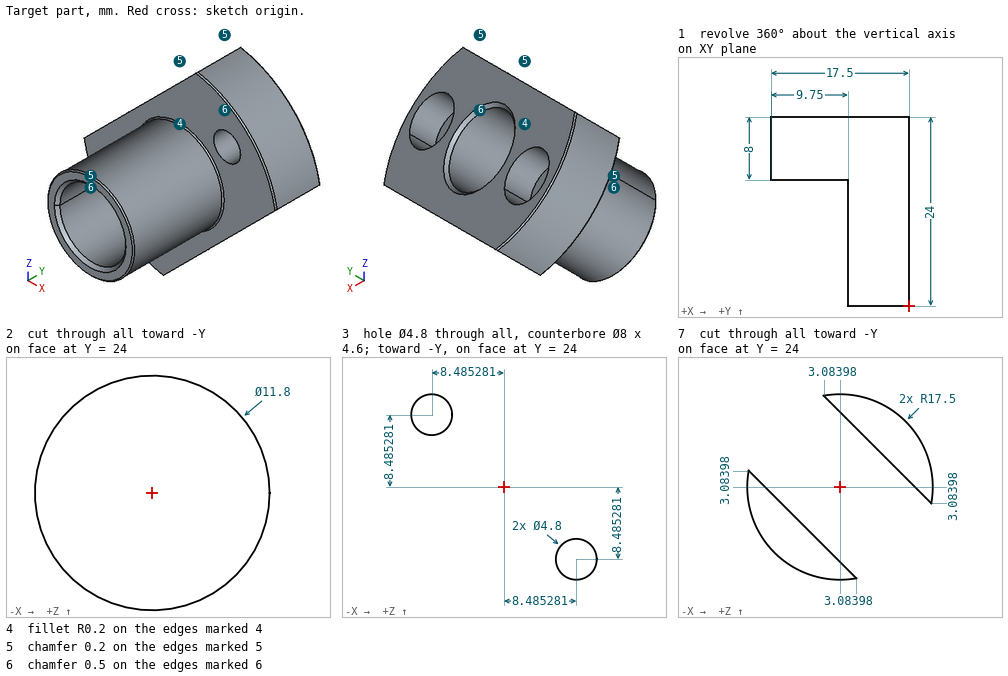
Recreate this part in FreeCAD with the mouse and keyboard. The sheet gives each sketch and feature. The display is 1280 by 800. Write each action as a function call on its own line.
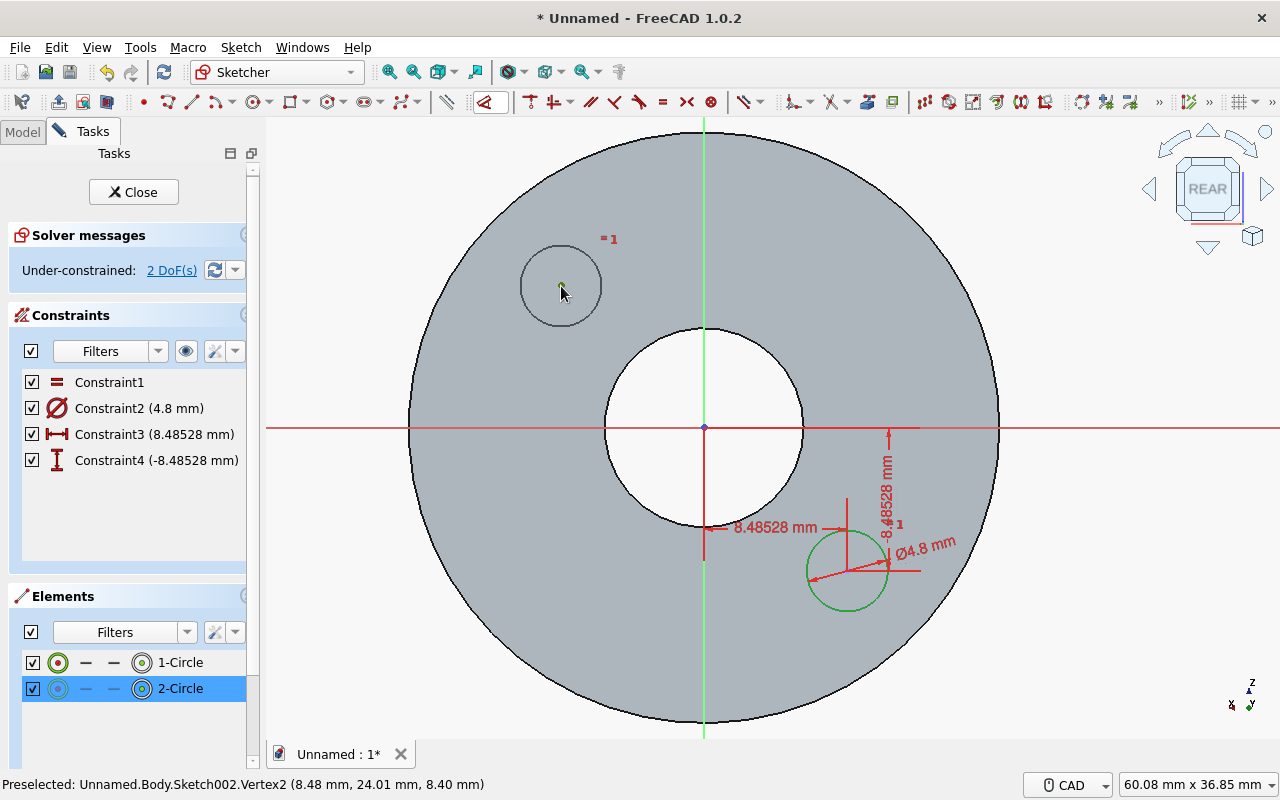
click(502, 102)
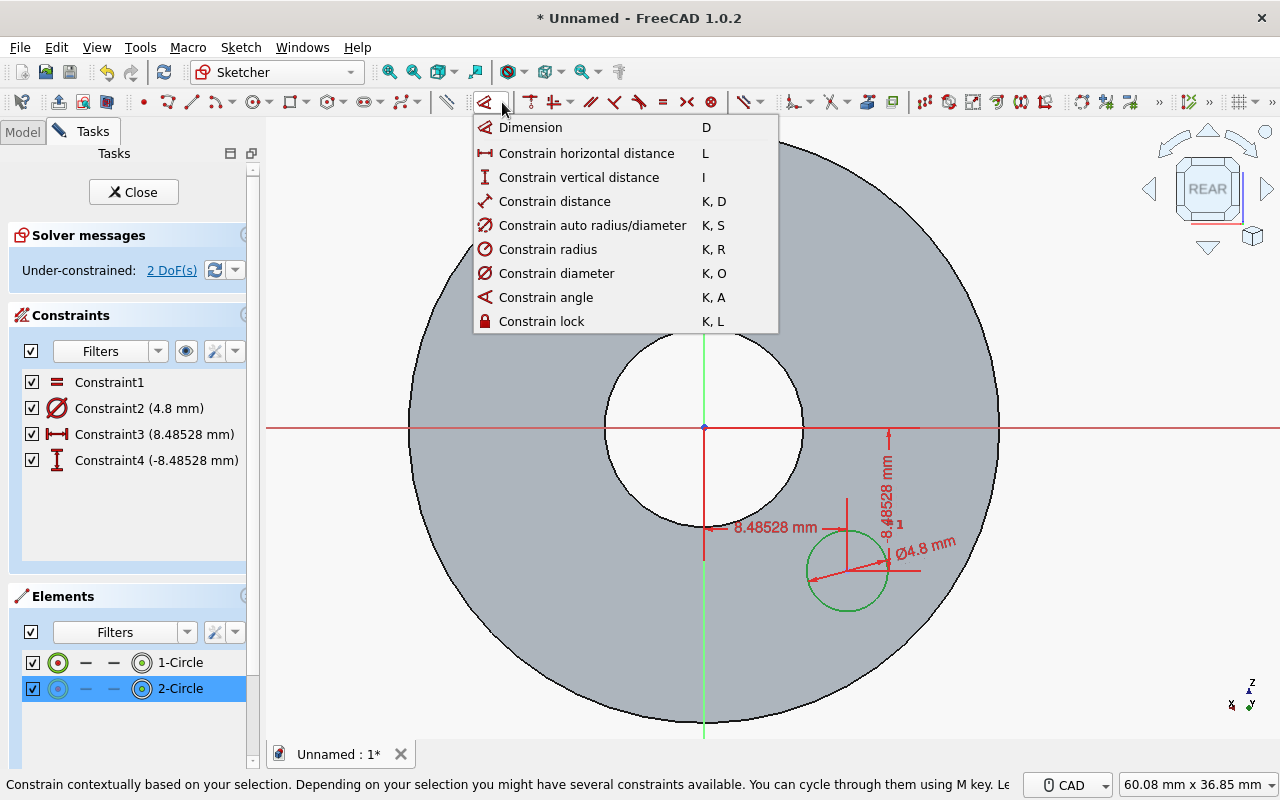
click(626, 153)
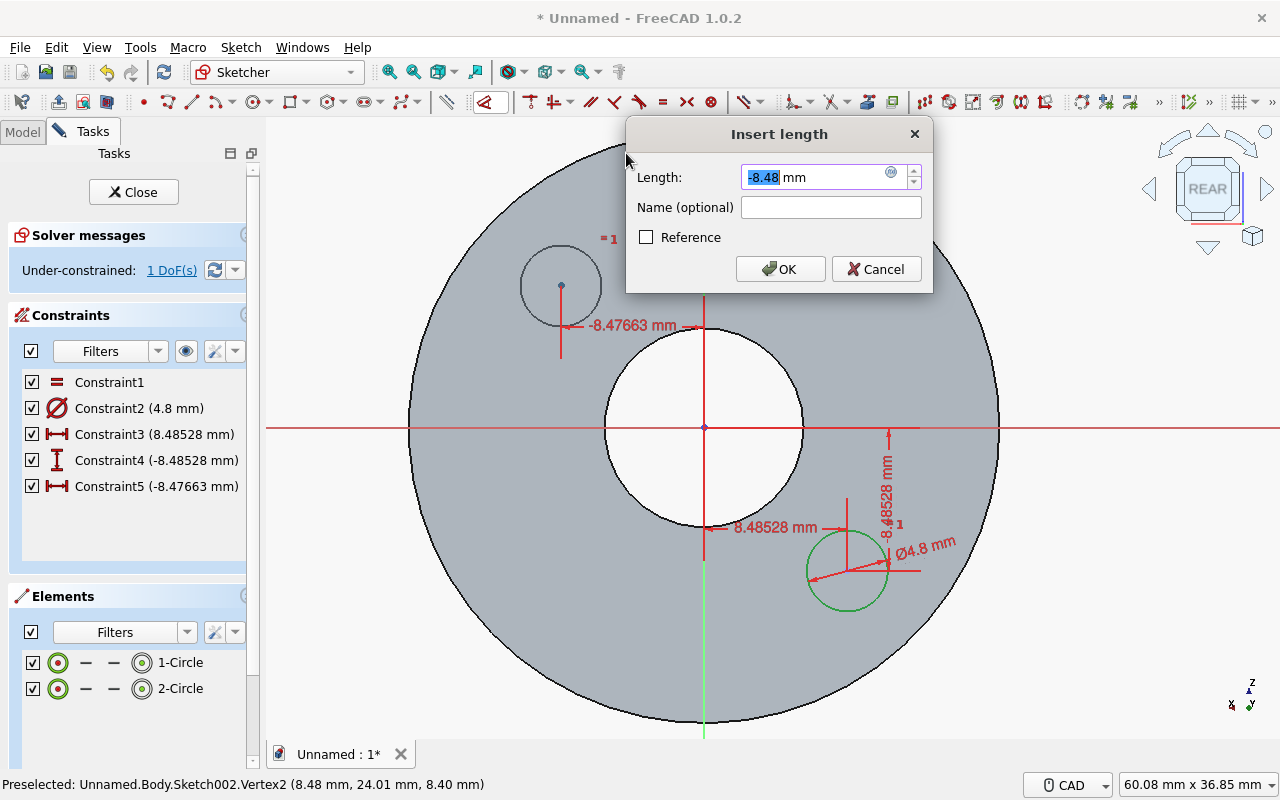
text(-8.485281)
key(Return)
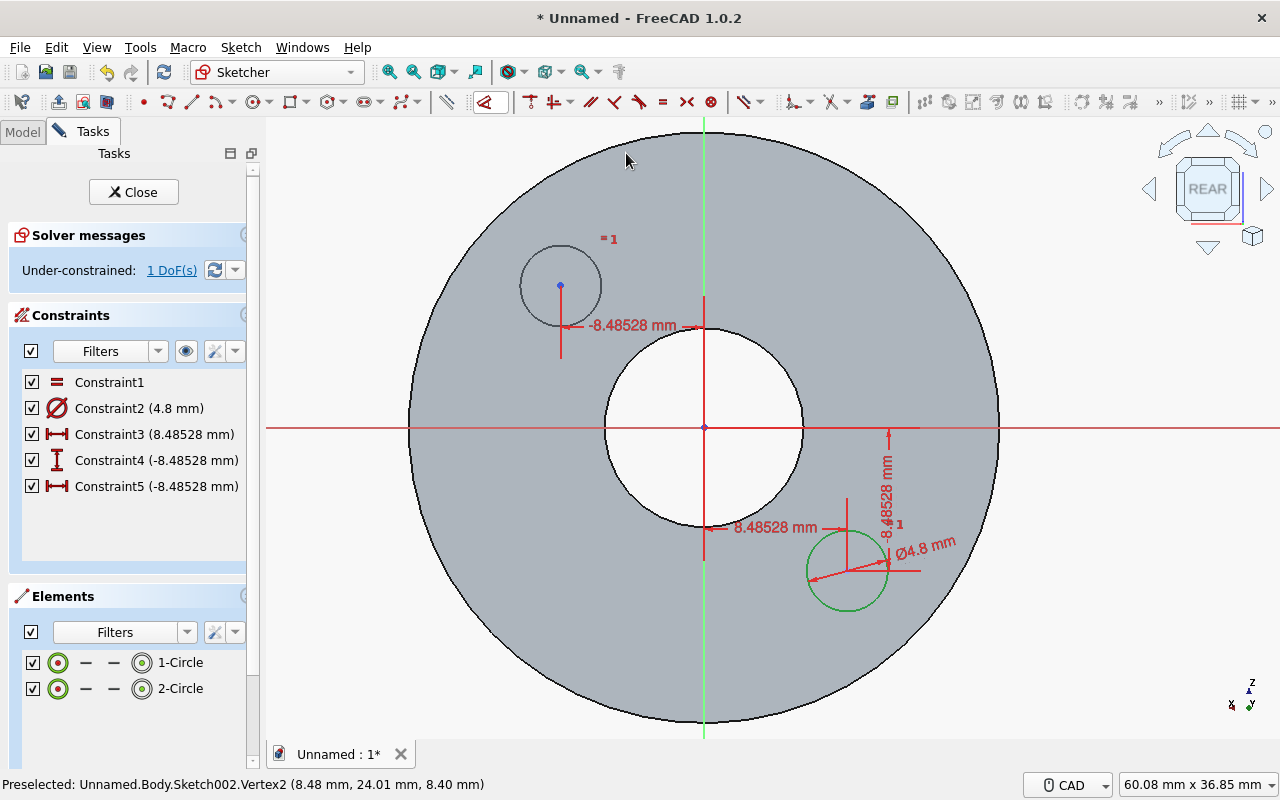
click(561, 286)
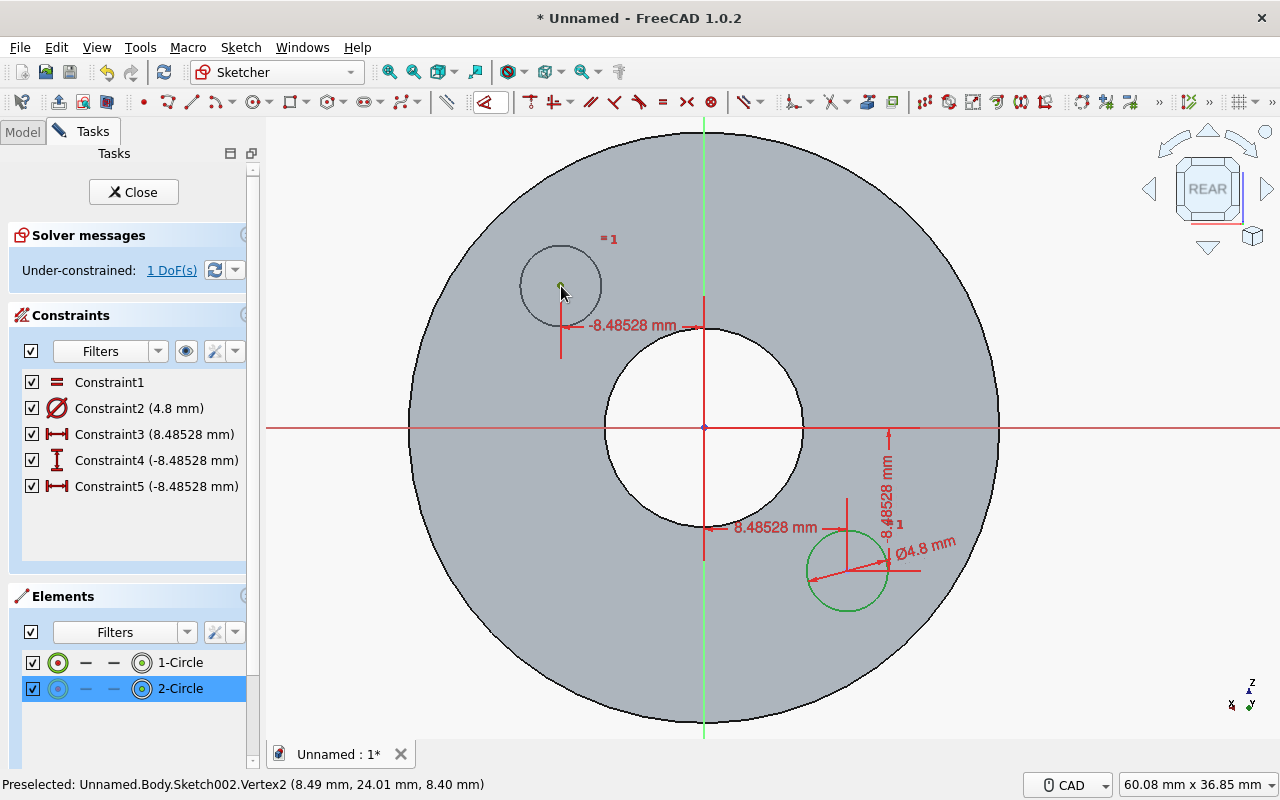
key(i)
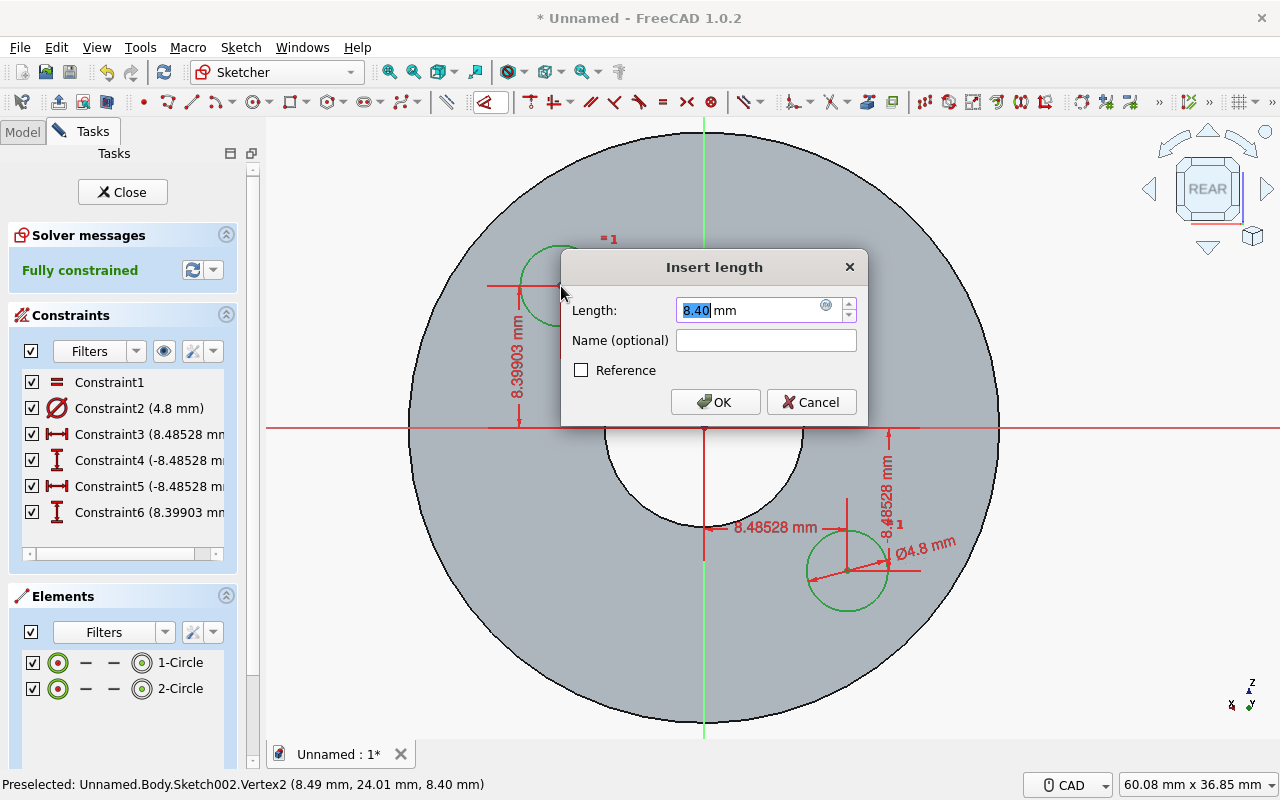
text(8.485281)
key(Return)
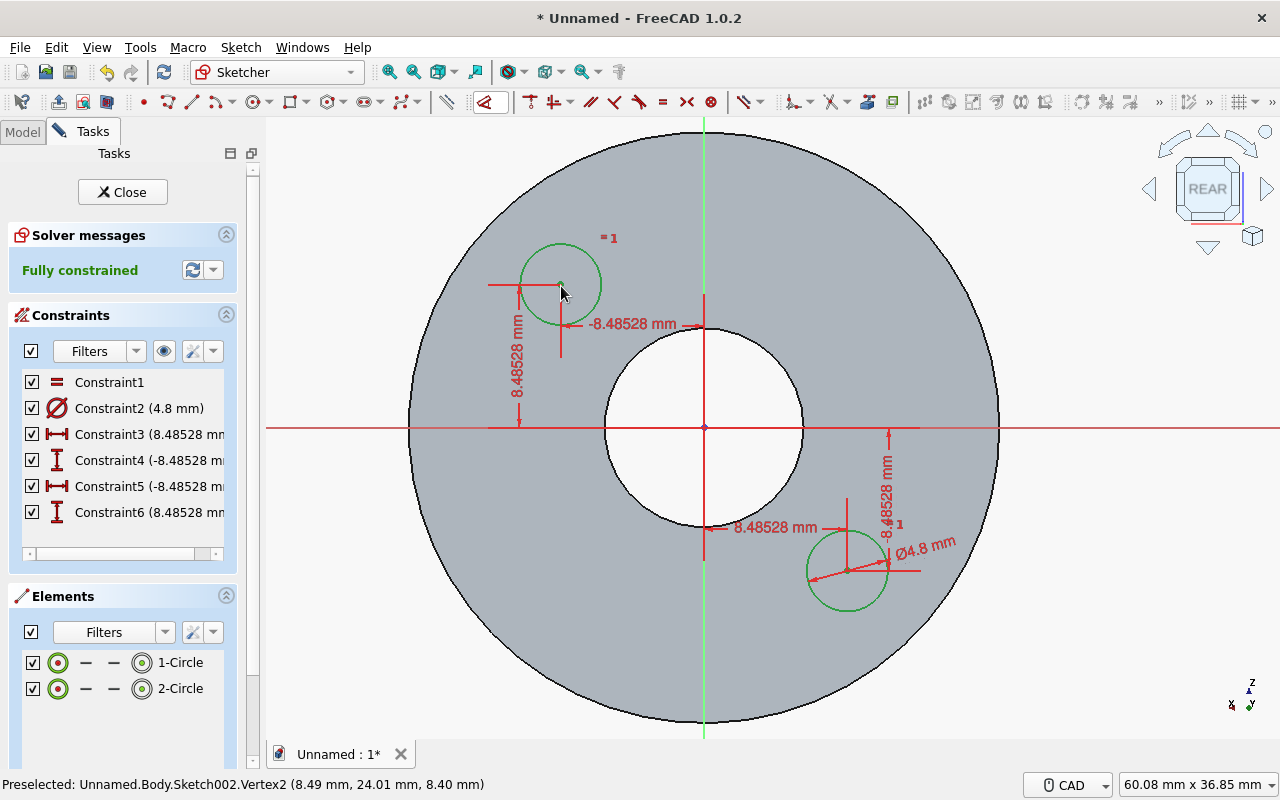
click(123, 192)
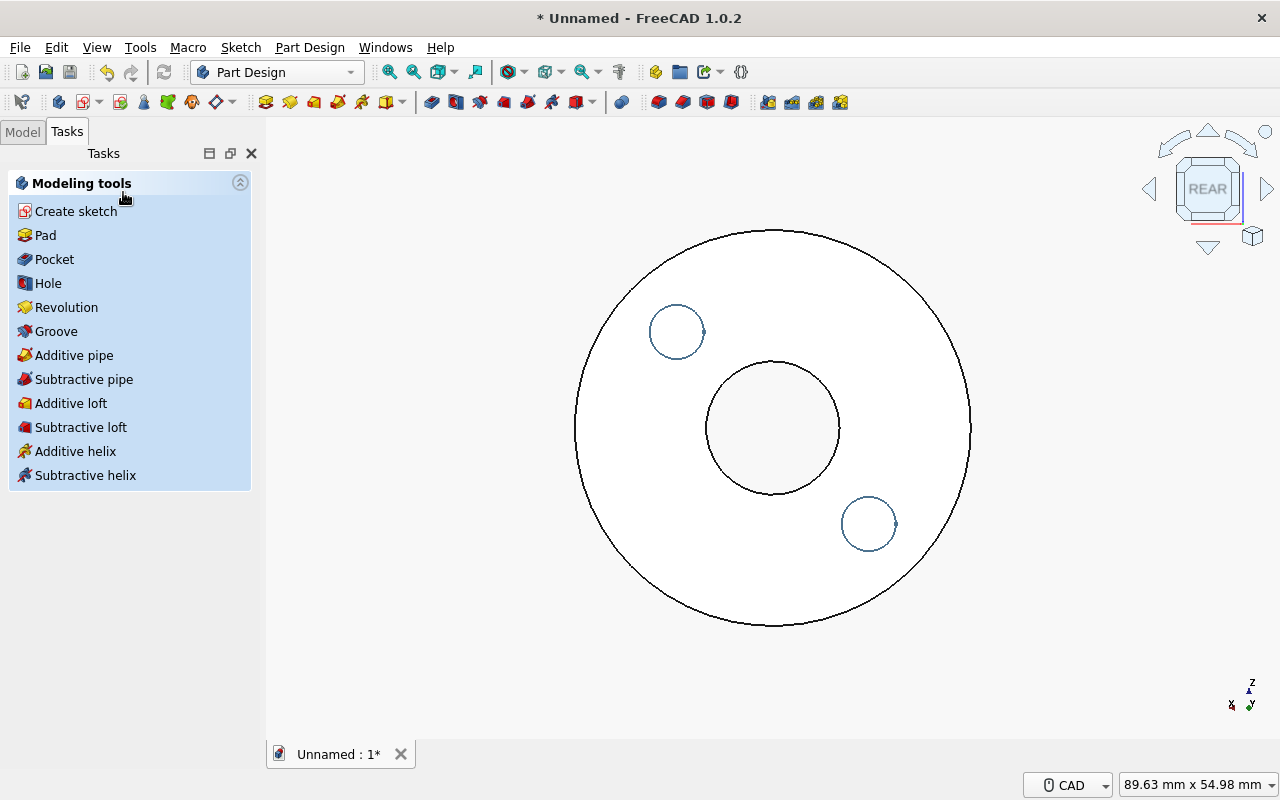
click(456, 102)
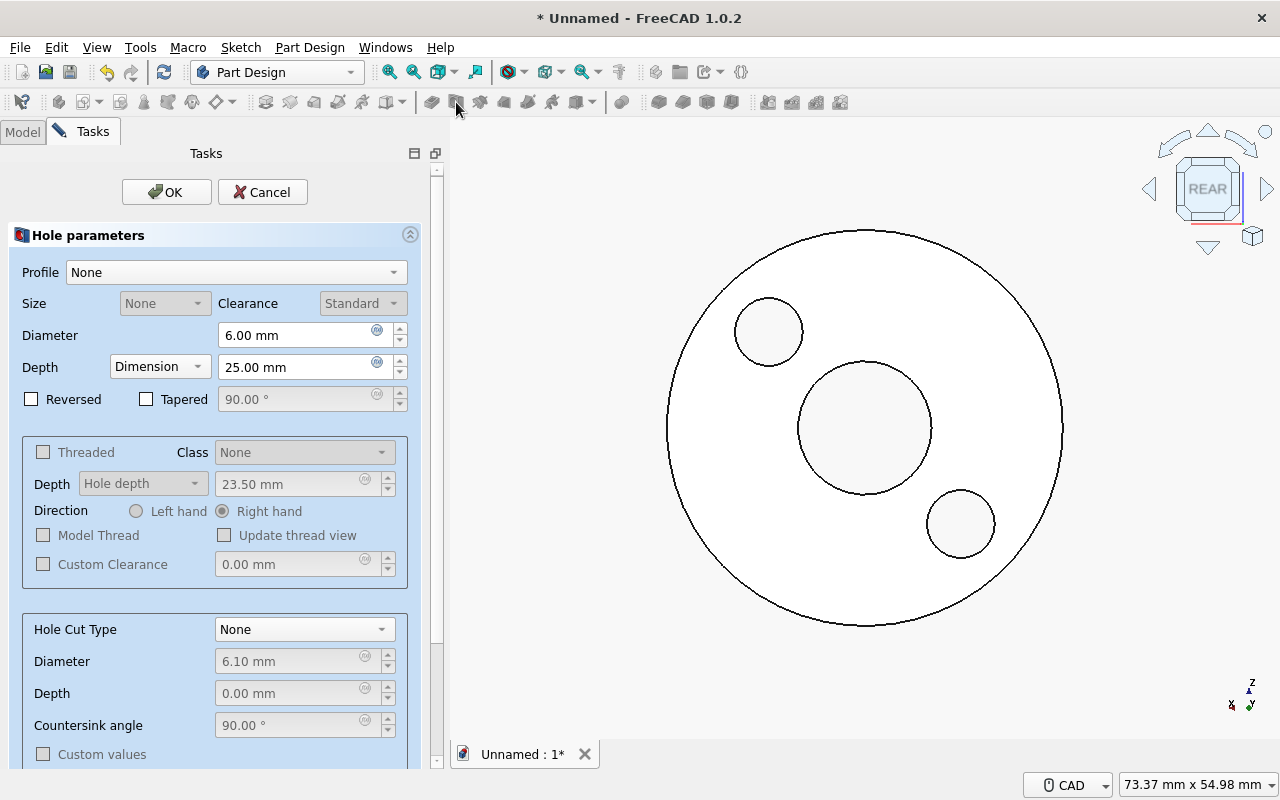
triple_click(305, 335)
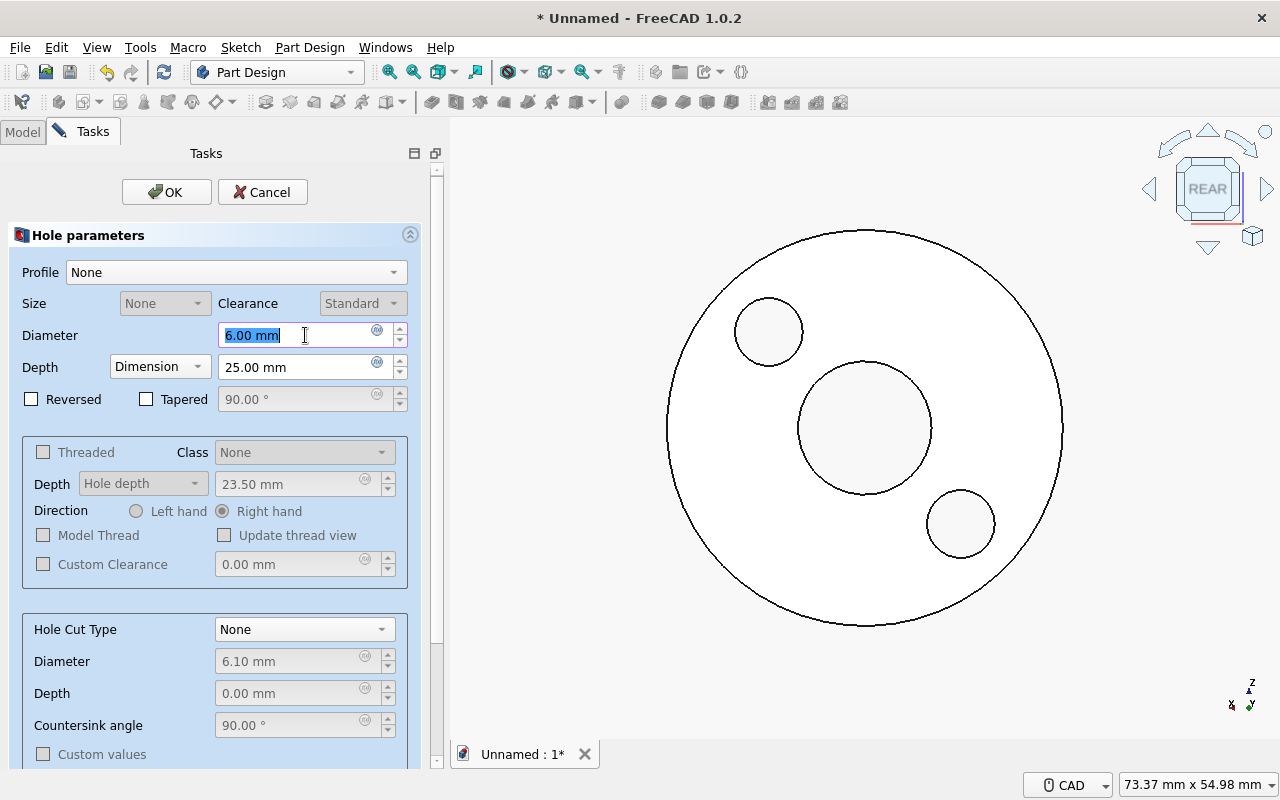
text(4.8)
key(Tab)